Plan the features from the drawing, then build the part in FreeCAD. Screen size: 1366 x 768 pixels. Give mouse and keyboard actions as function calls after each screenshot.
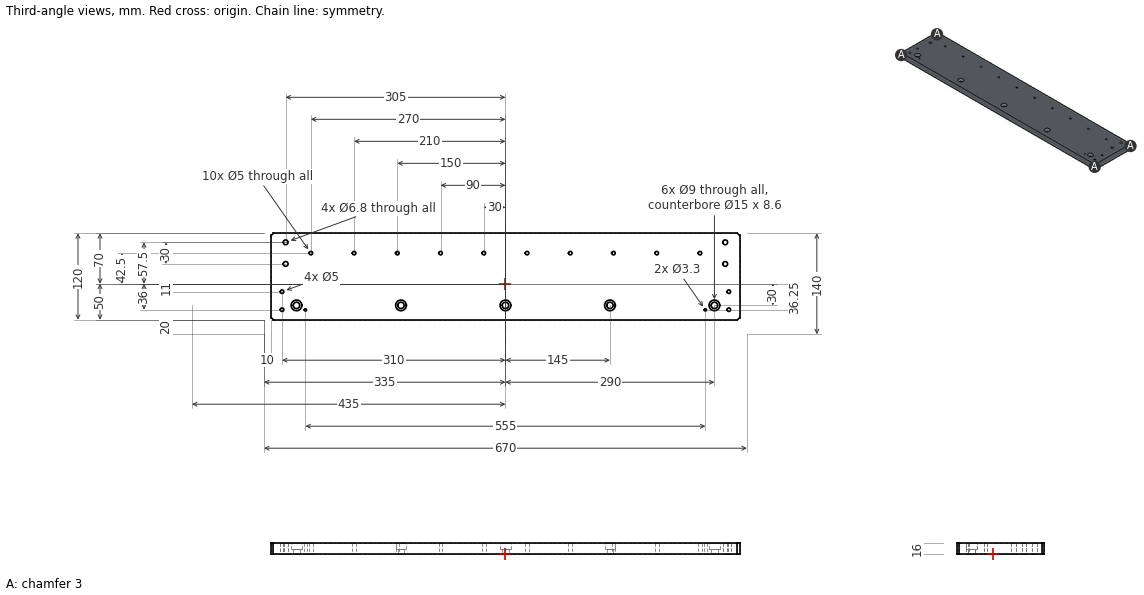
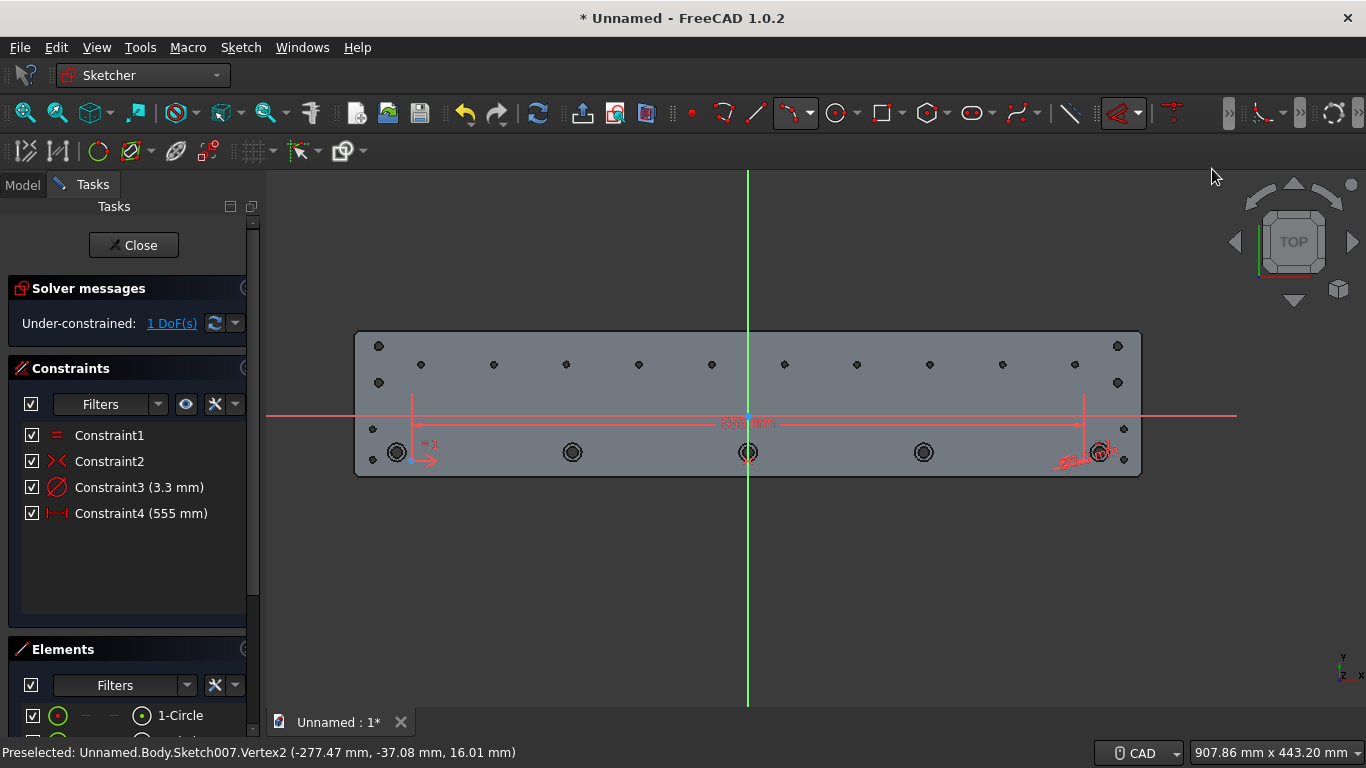
click(1084, 461)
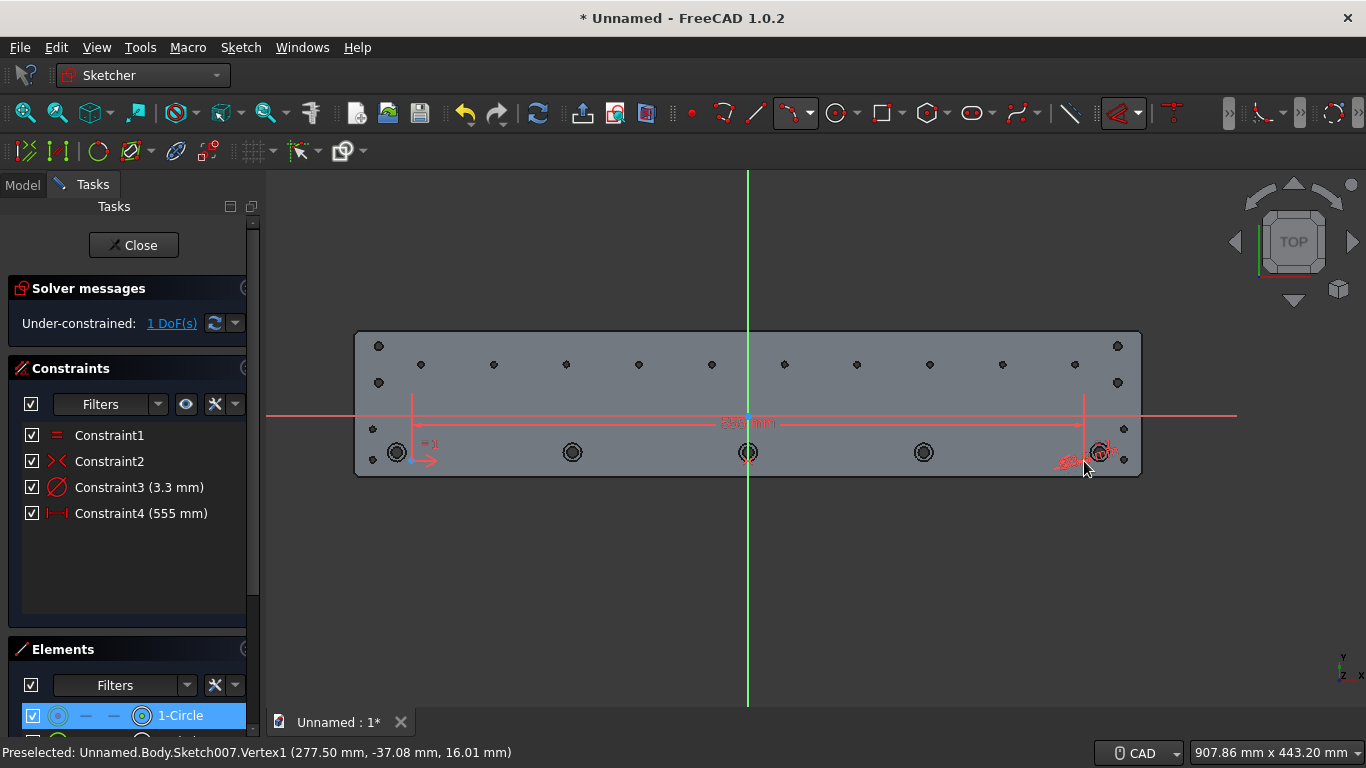
click(1140, 114)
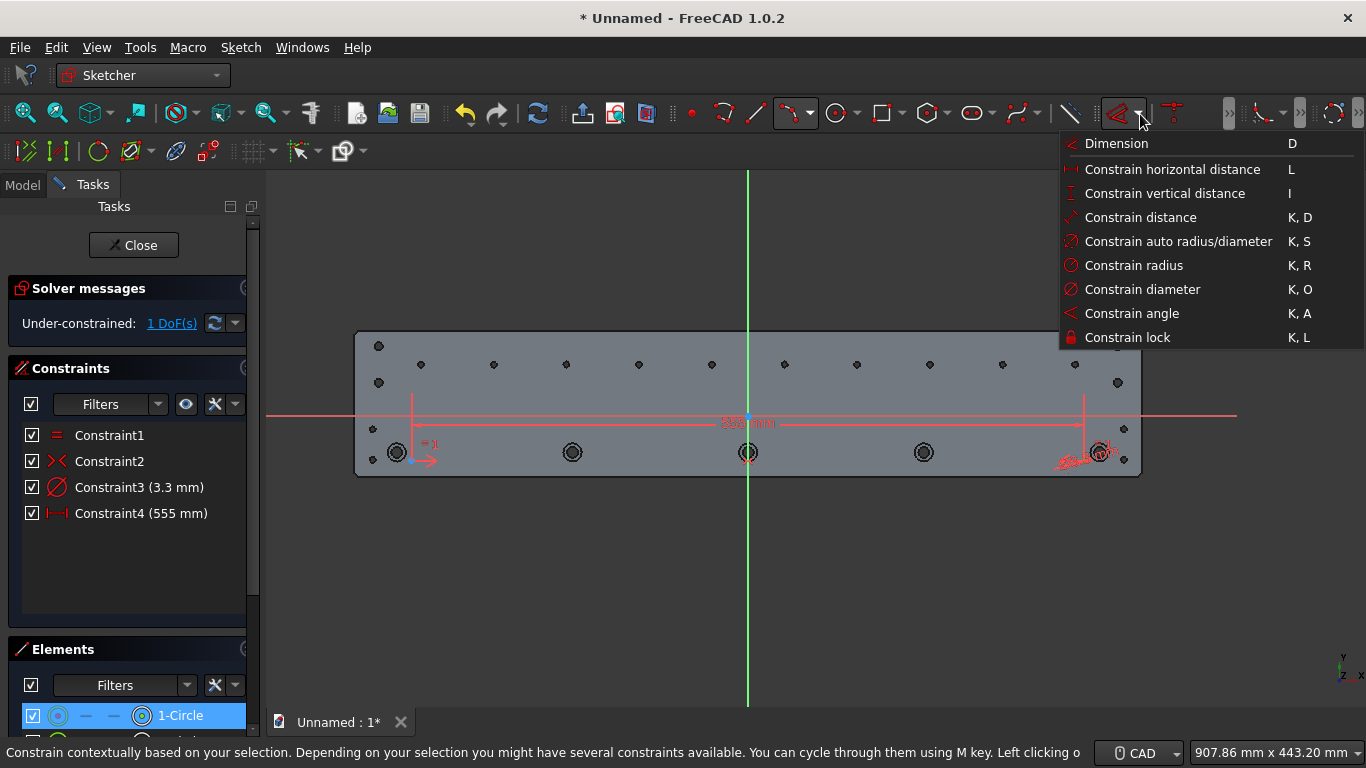
click(1212, 193)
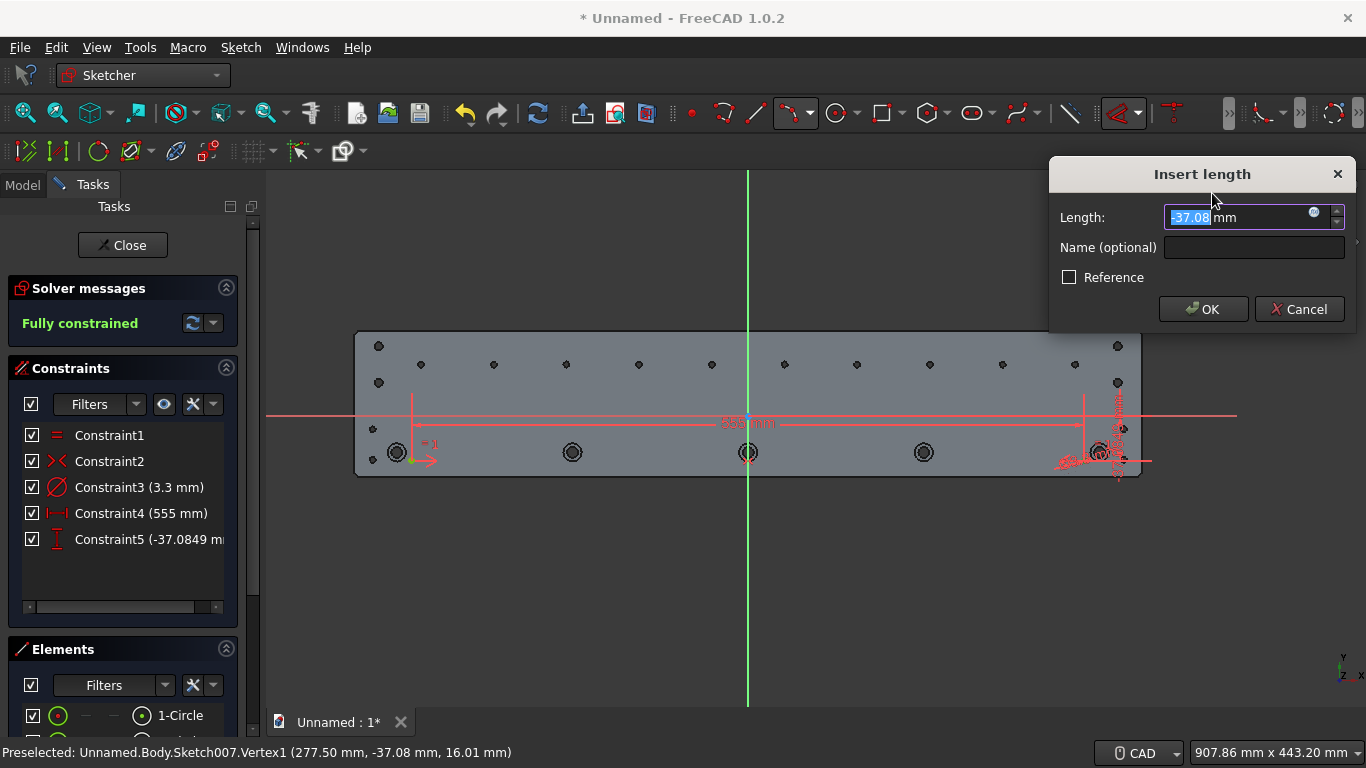
text(-36.25)
key(Return)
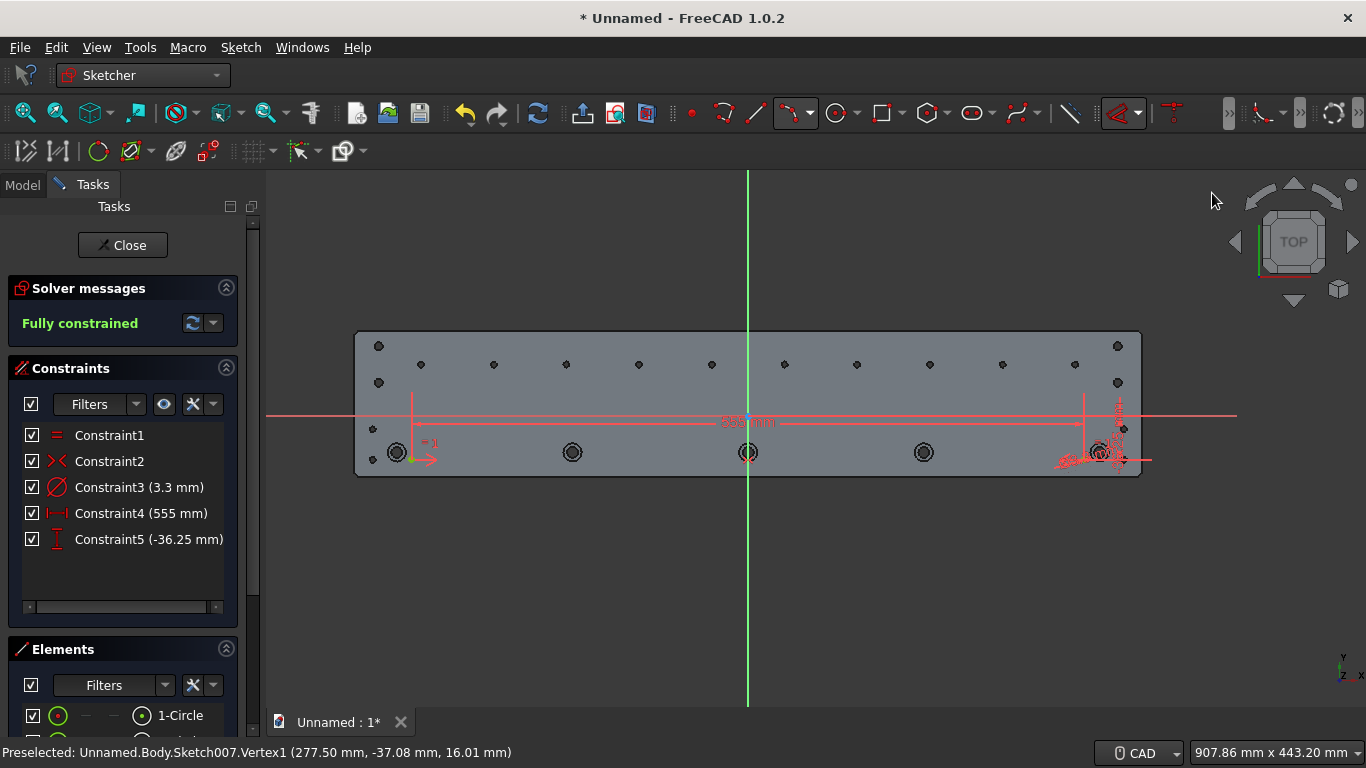
click(123, 245)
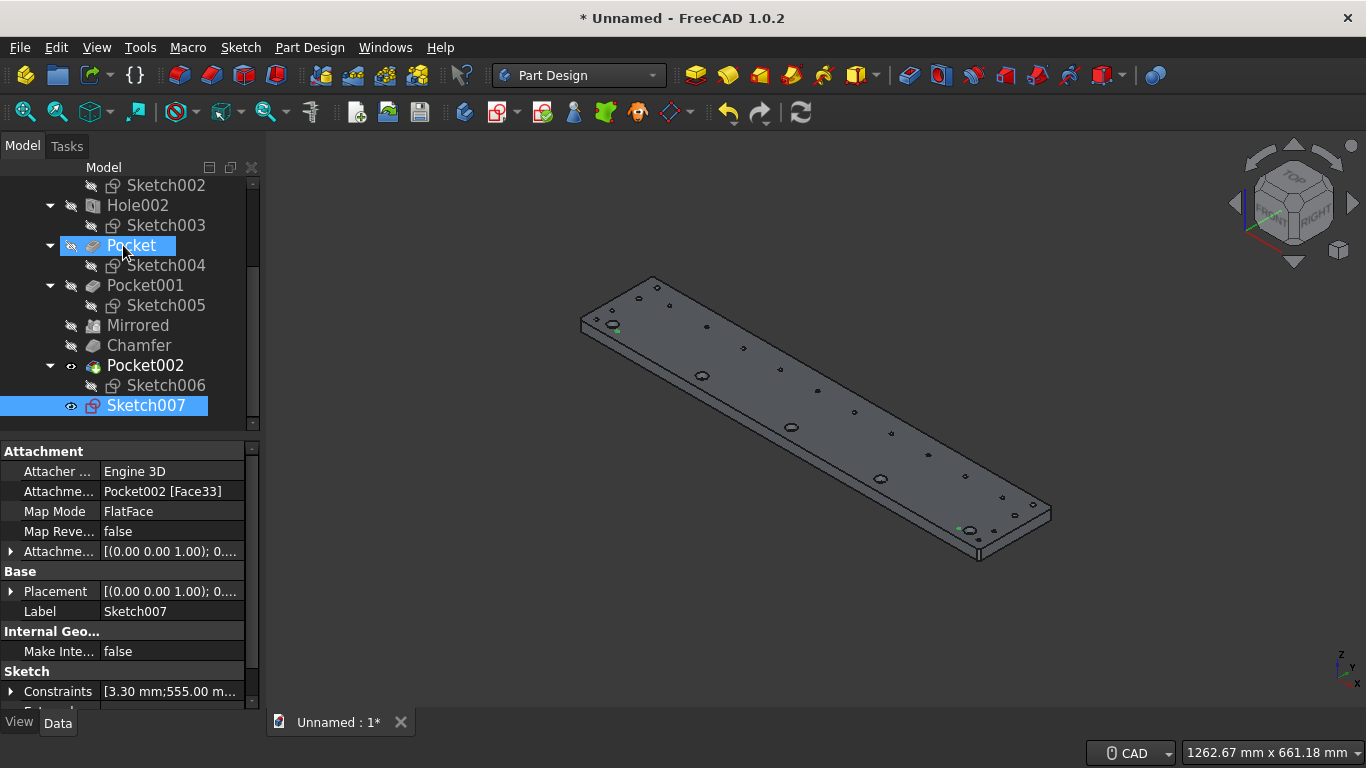
click(910, 76)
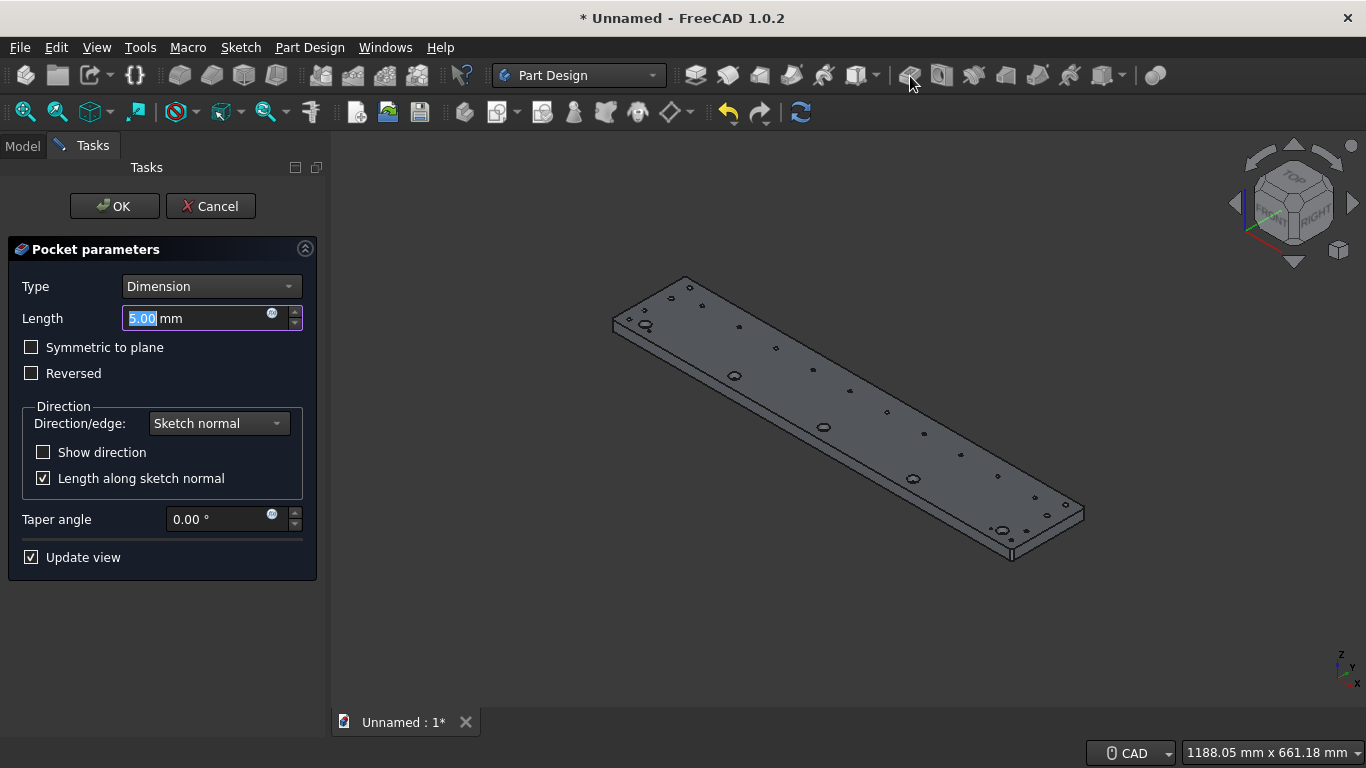
click(212, 286)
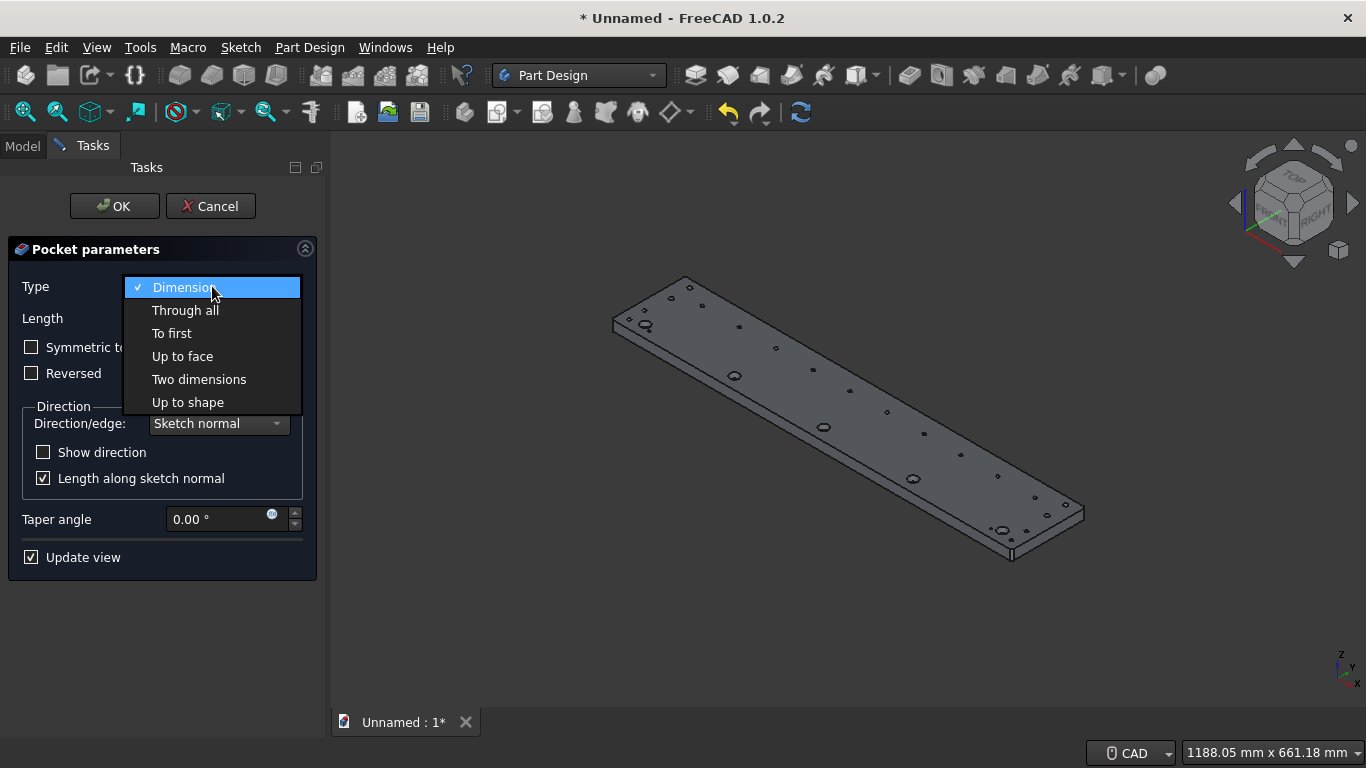
click(212, 310)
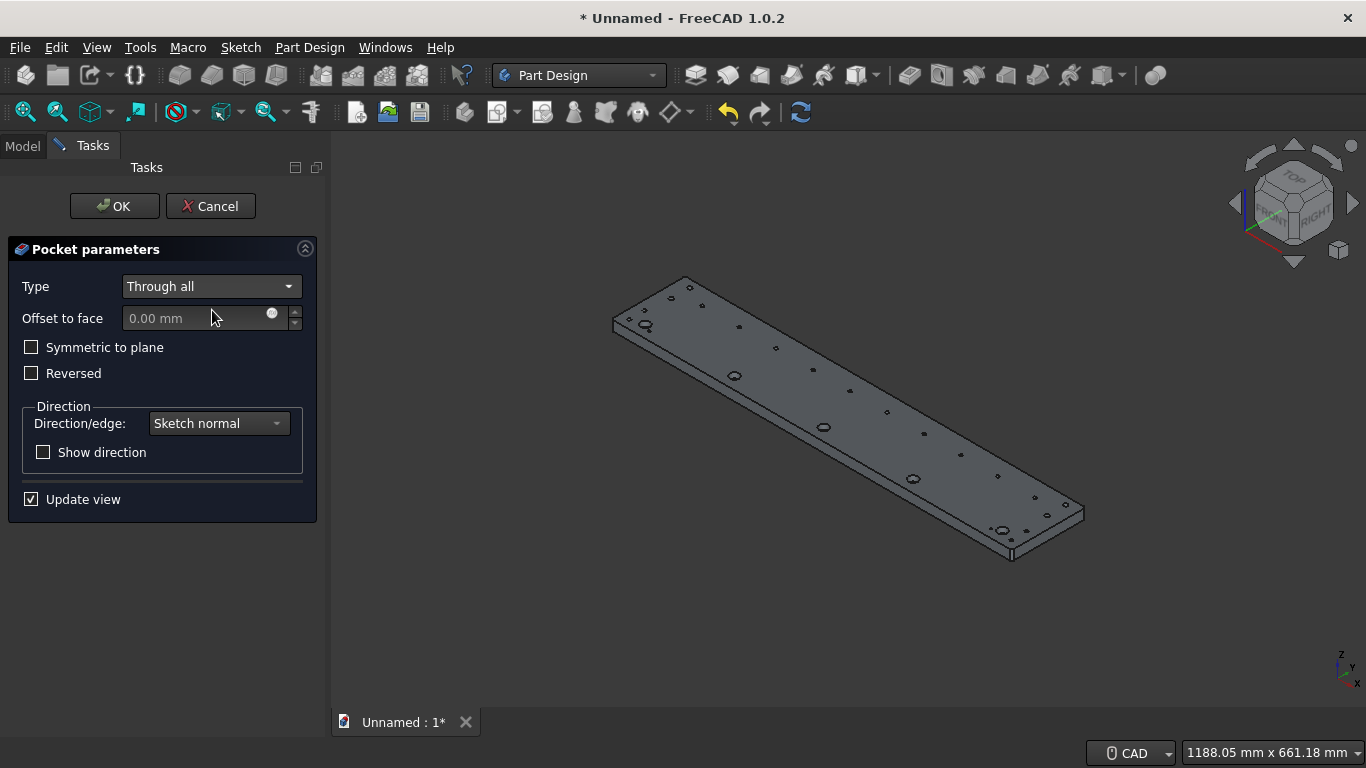
click(115, 206)